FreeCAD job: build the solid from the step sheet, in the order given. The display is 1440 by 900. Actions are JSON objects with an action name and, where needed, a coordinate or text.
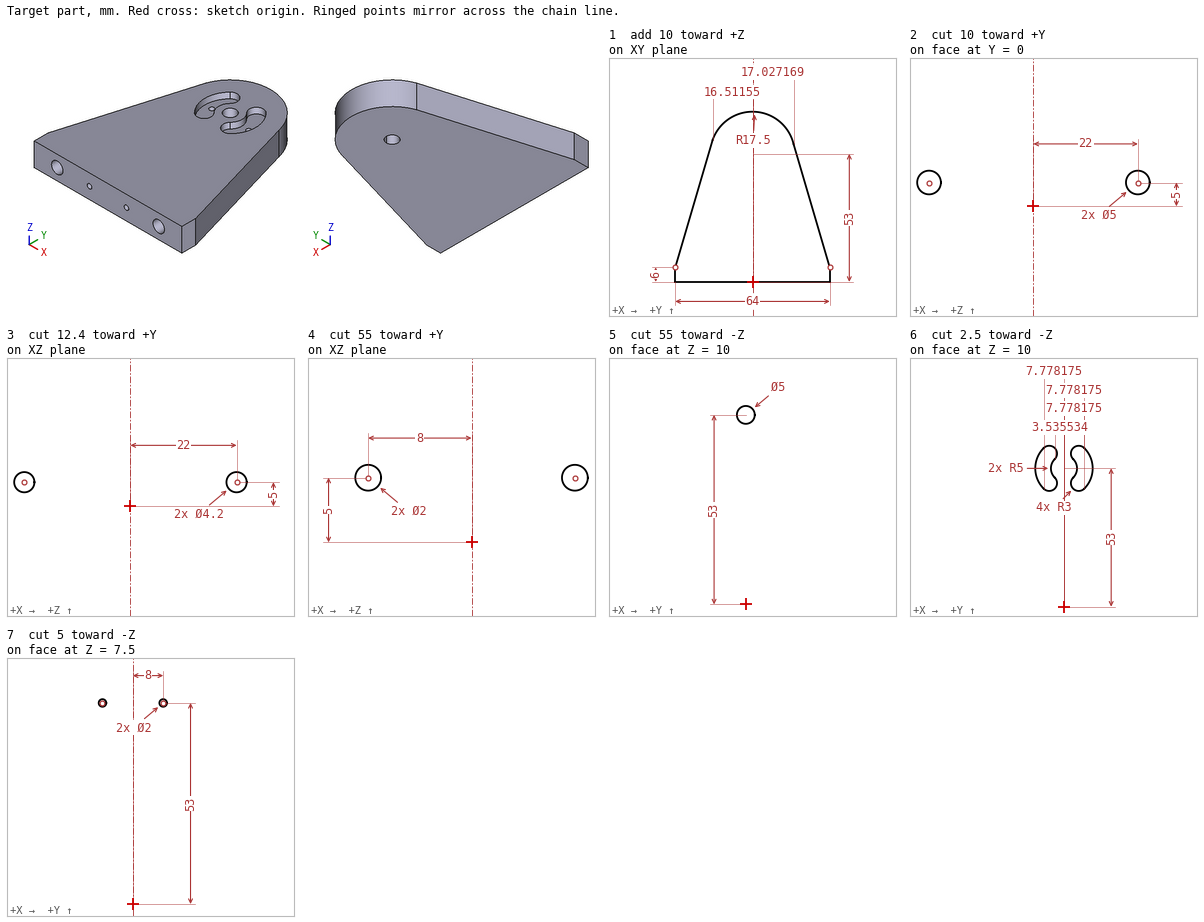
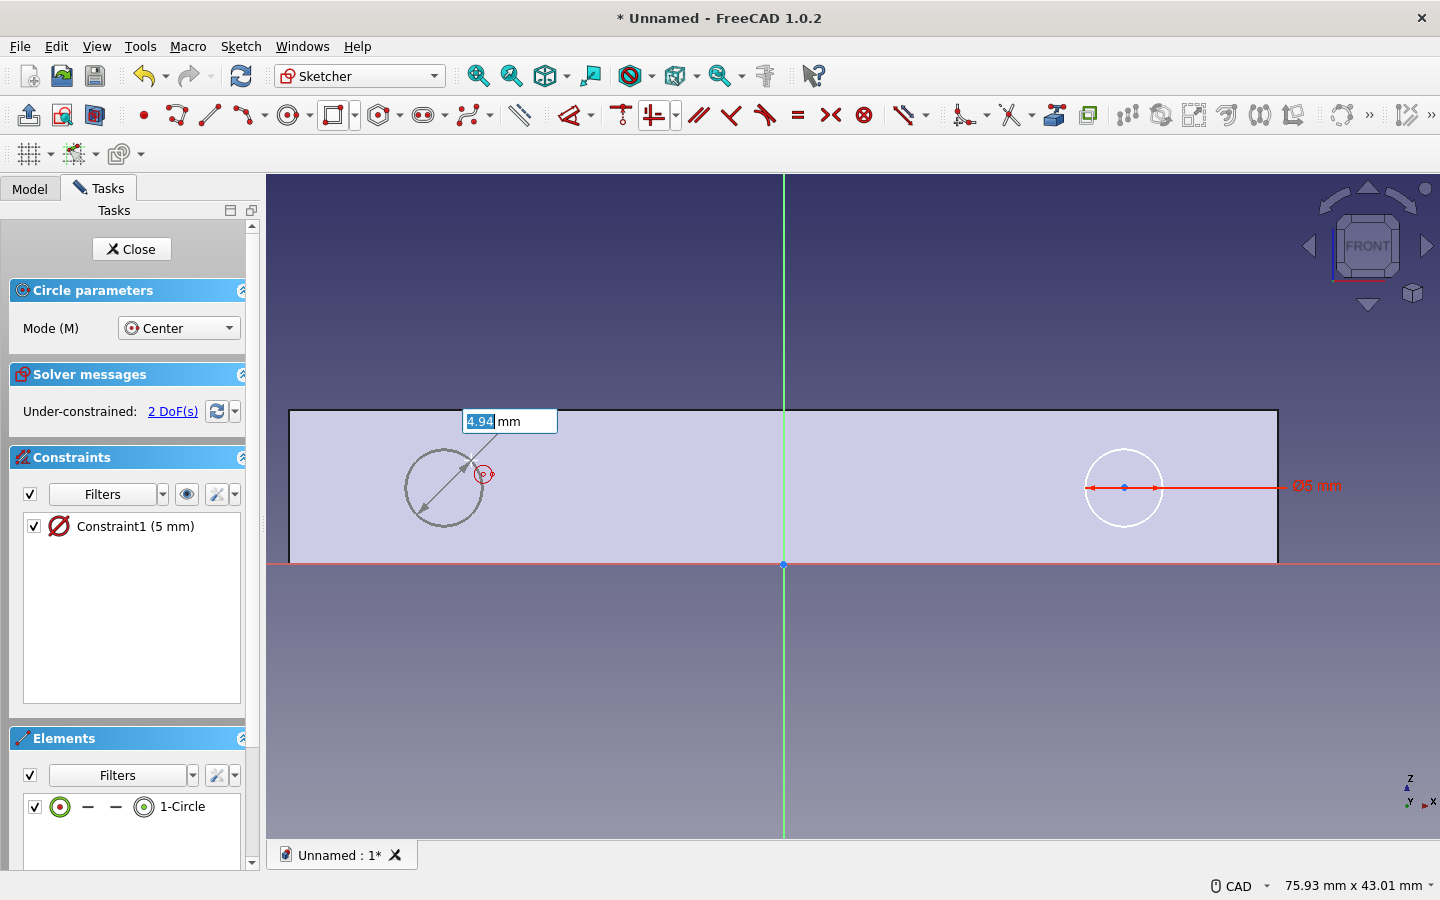
{"action": "type", "text": "5"}
{"action": "key", "text": "Return"}
{"action": "key", "text": "Escape"}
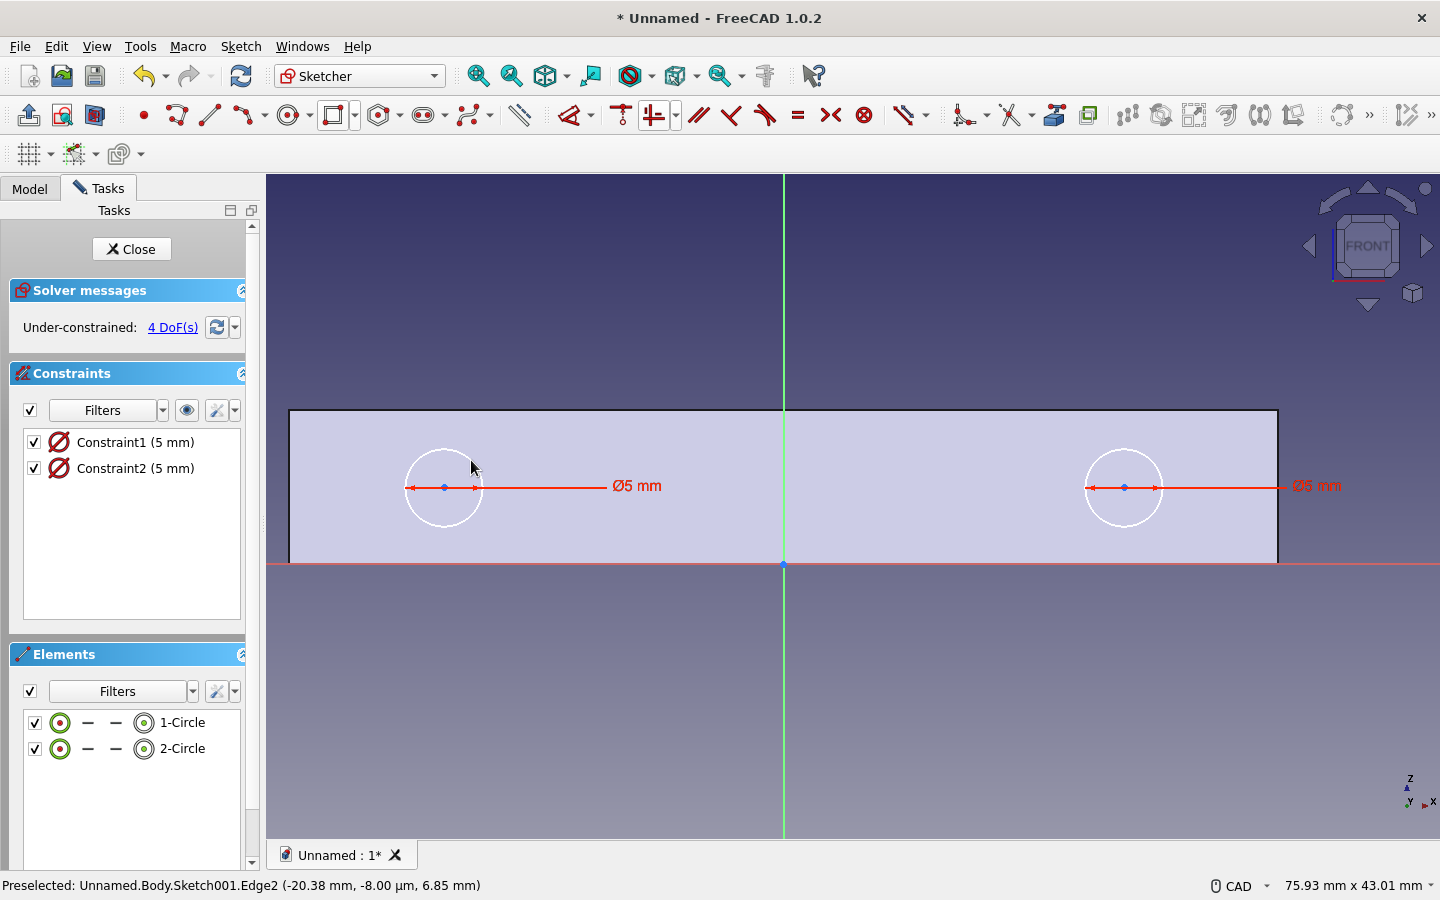
{"action": "left_click", "coordinate": [1124, 488]}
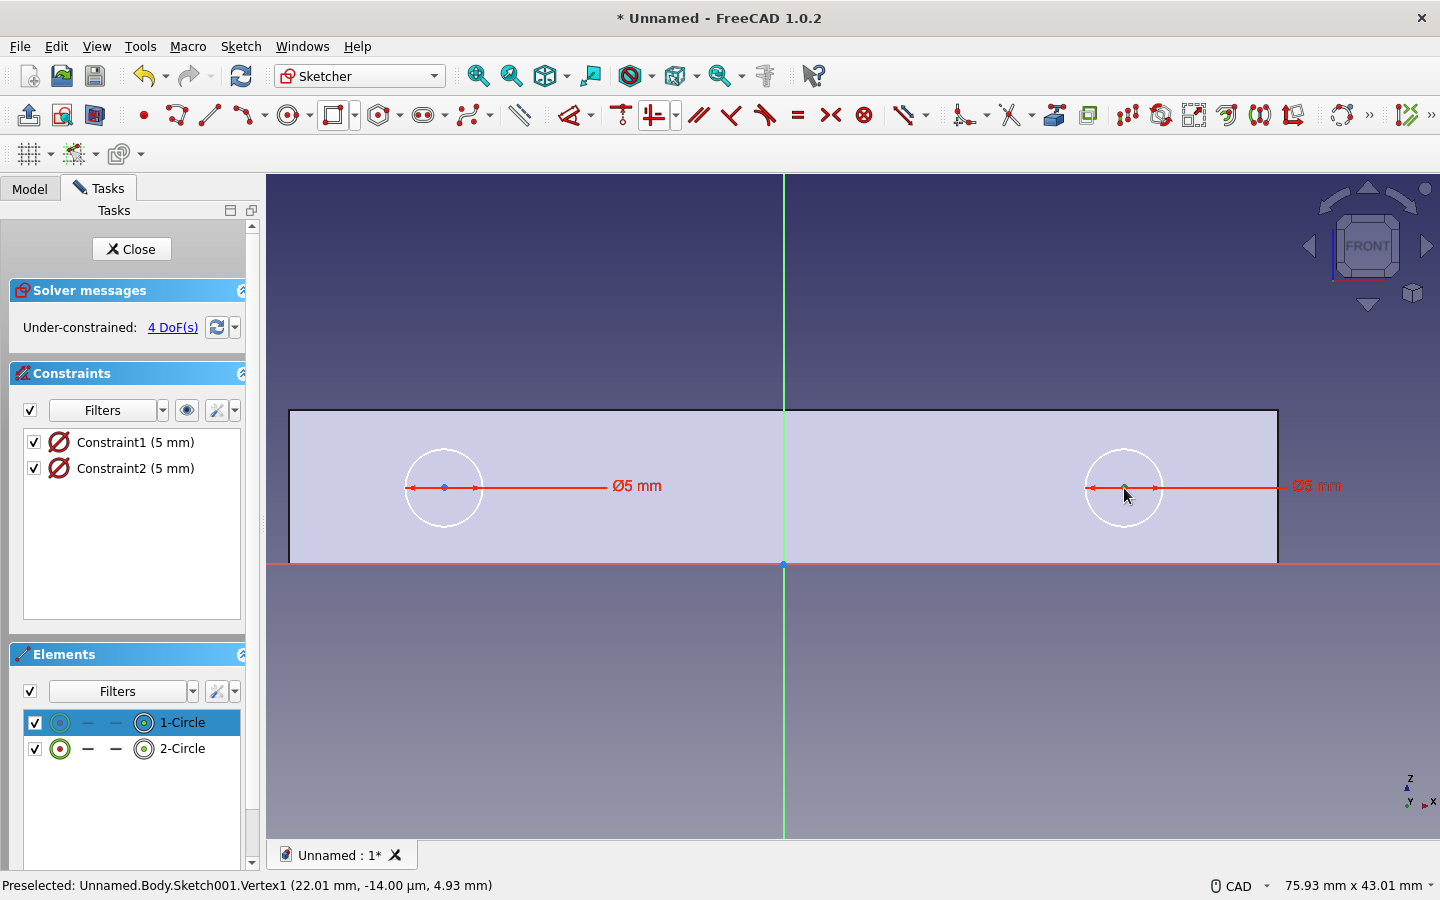
{"action": "left_click", "coordinate": [444, 488]}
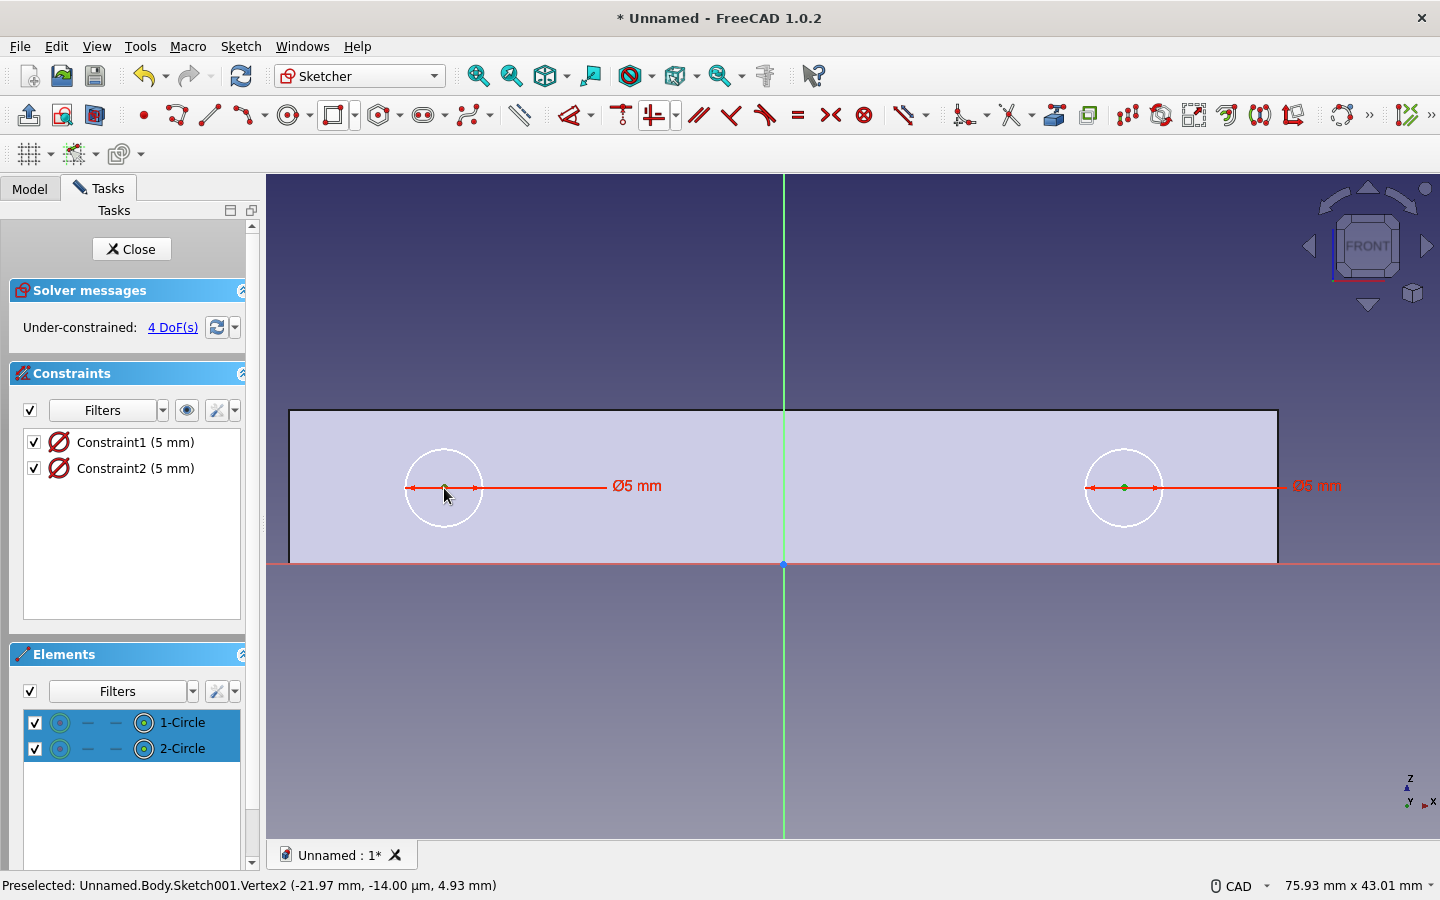
{"action": "left_click", "coordinate": [784, 768]}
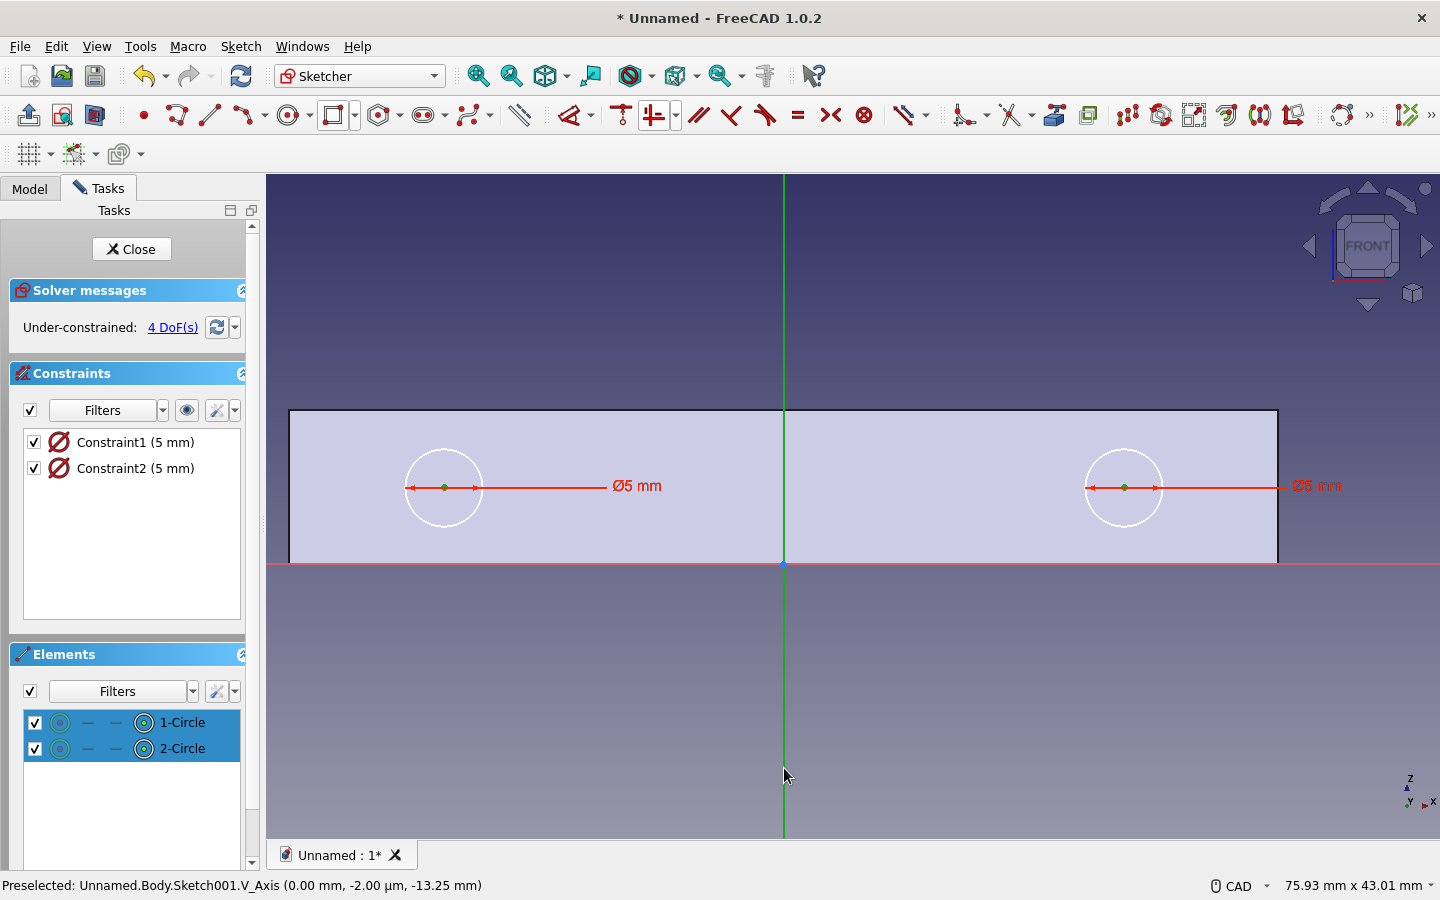
{"action": "left_click", "coordinate": [831, 116]}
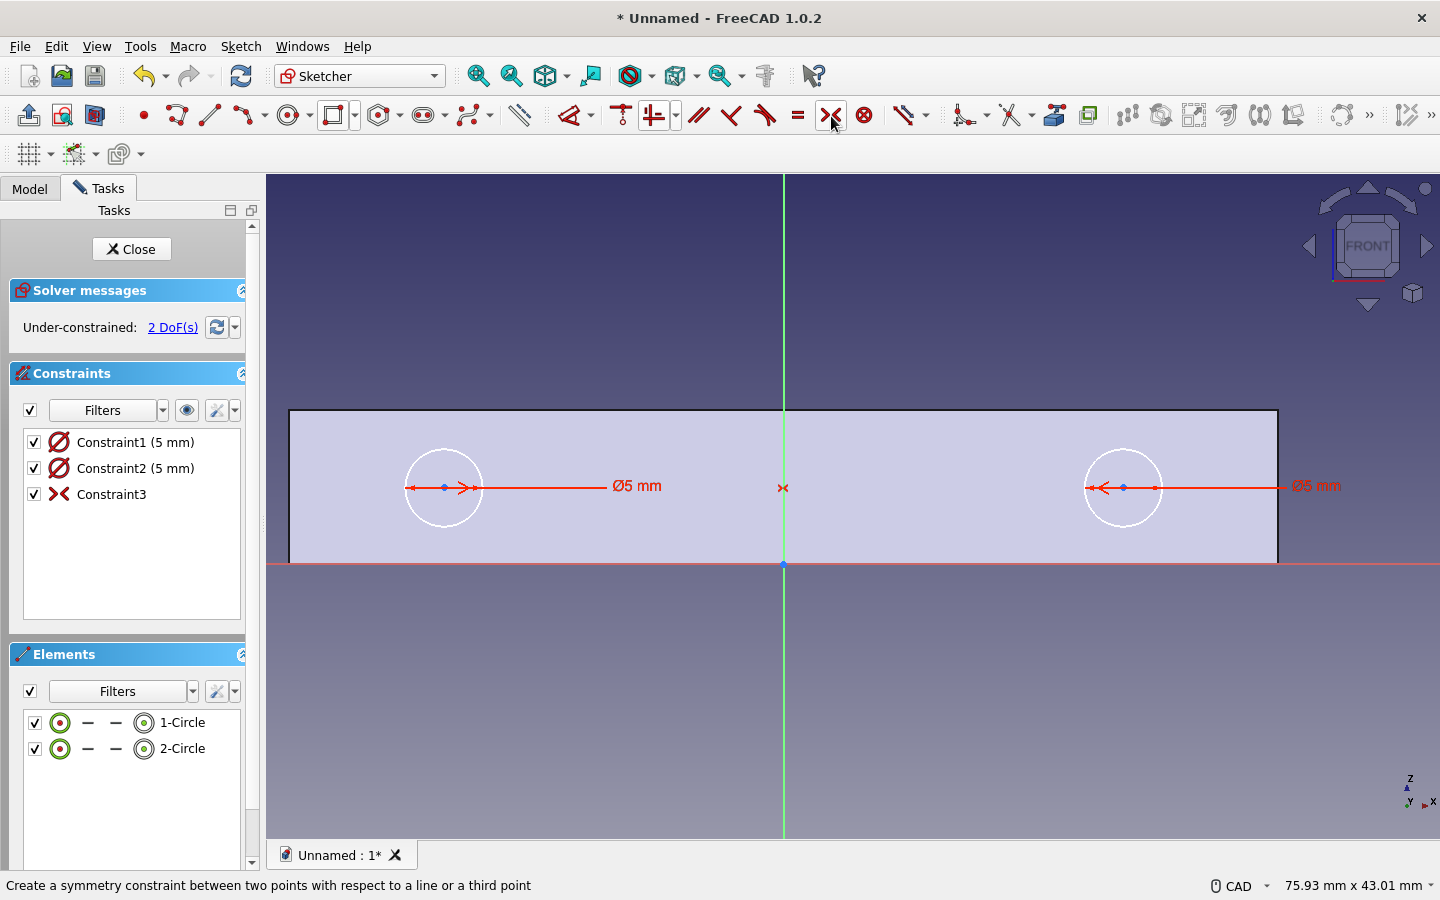
{"action": "key", "text": "d"}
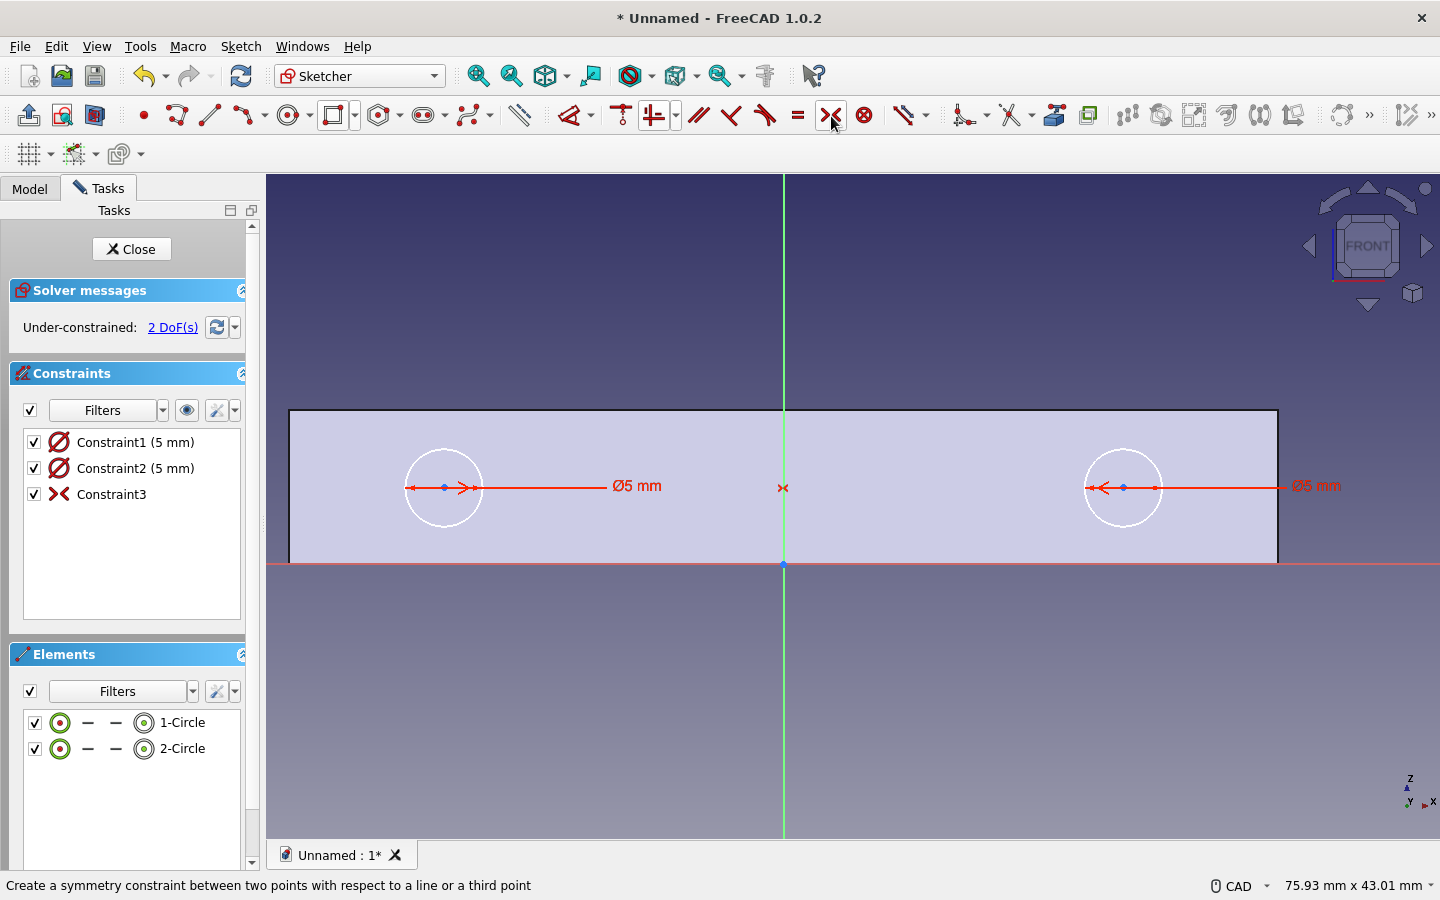
{"action": "left_click", "coordinate": [1123, 488]}
{"action": "left_click", "coordinate": [1157, 544]}